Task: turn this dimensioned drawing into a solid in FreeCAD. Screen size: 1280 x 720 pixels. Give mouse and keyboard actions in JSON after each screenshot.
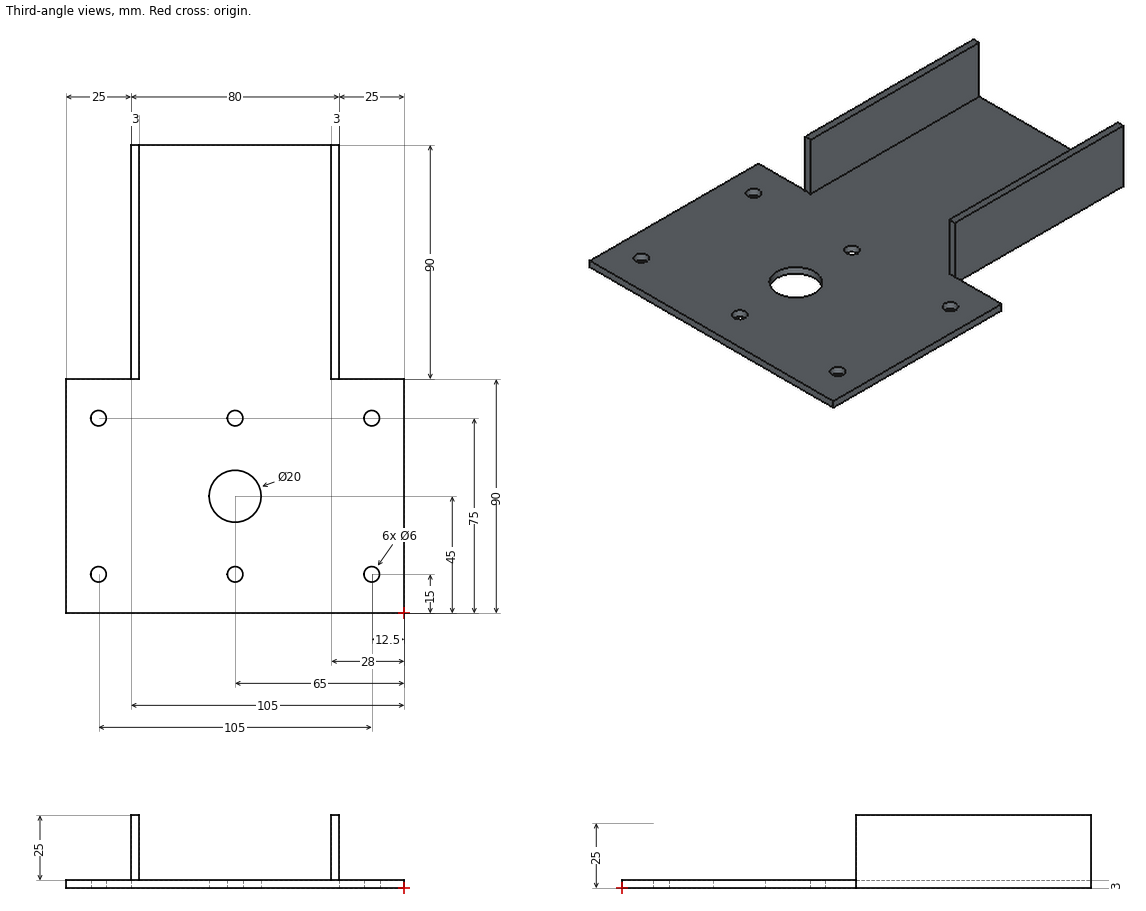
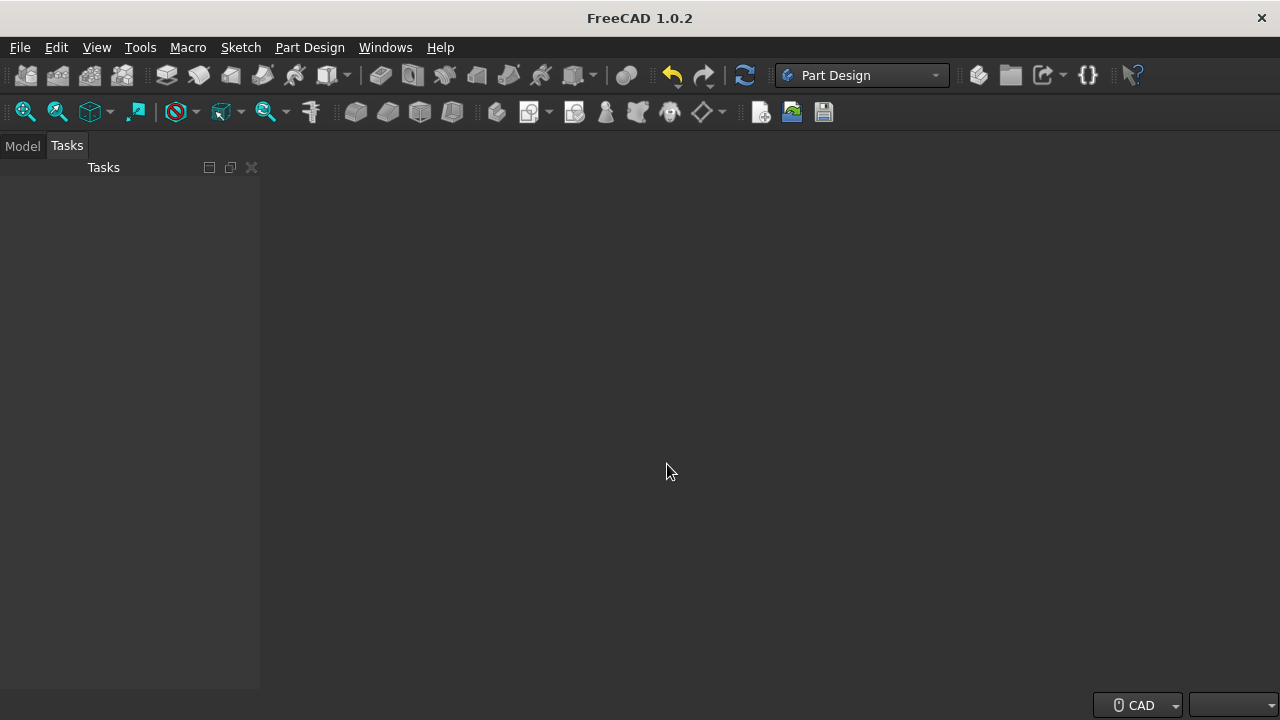
{"action": "left_click", "coordinate": [760, 112]}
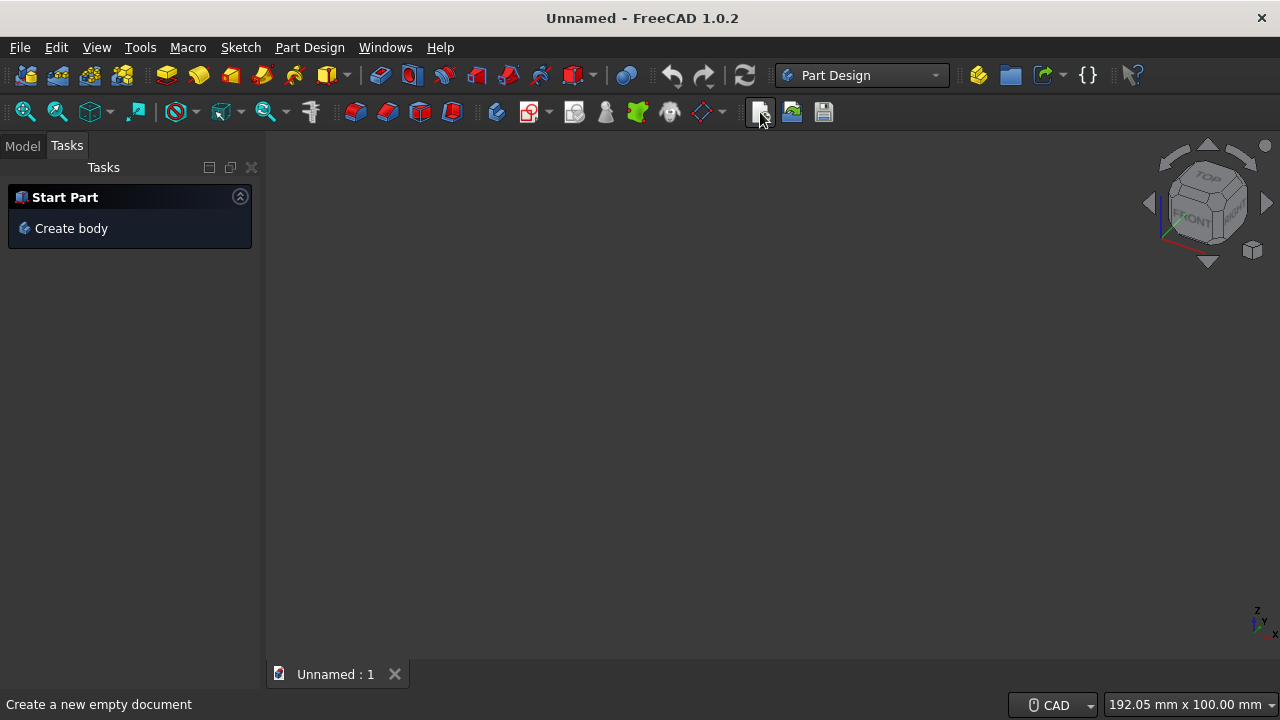
{"action": "left_click", "coordinate": [530, 112]}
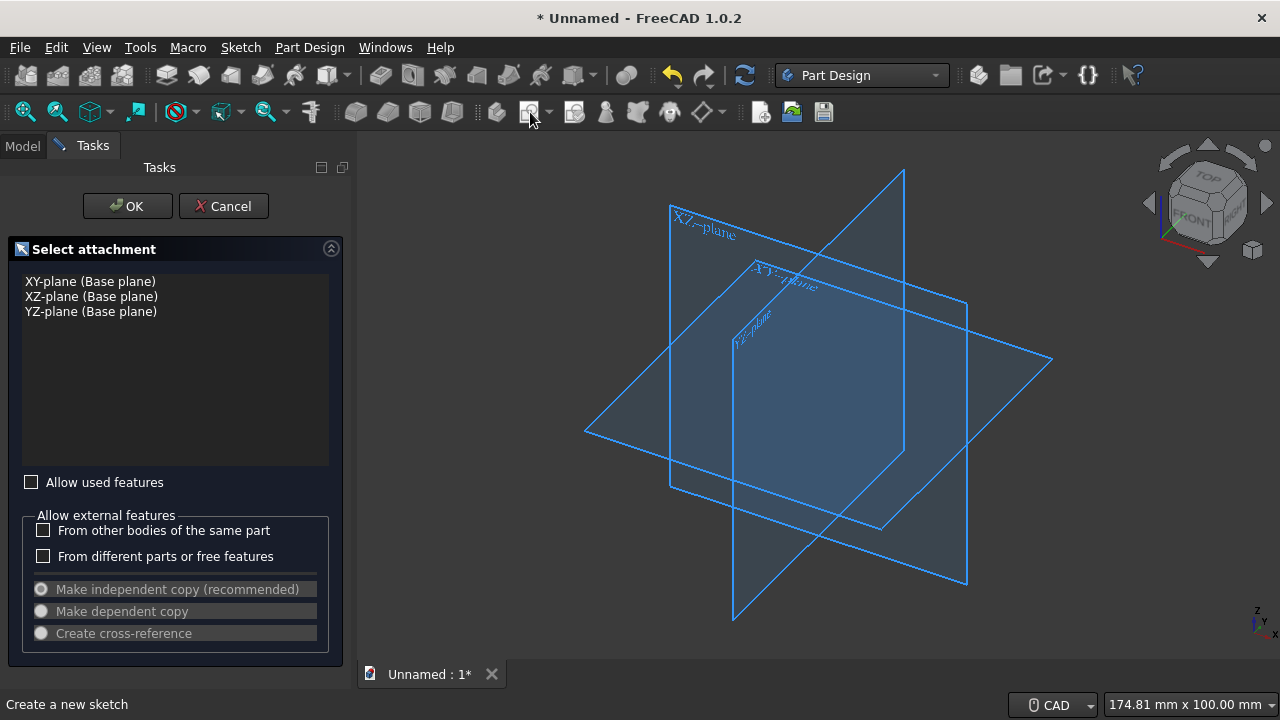
{"action": "left_click", "coordinate": [82, 282]}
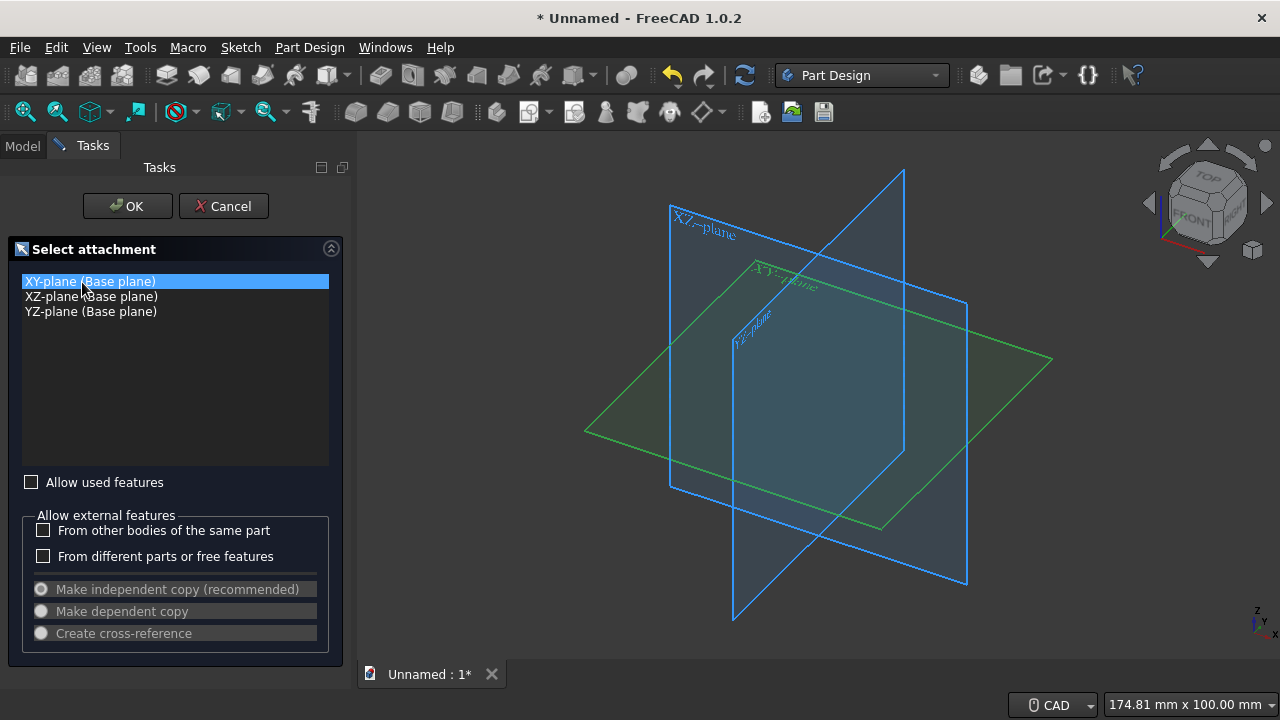
{"action": "left_click", "coordinate": [128, 206]}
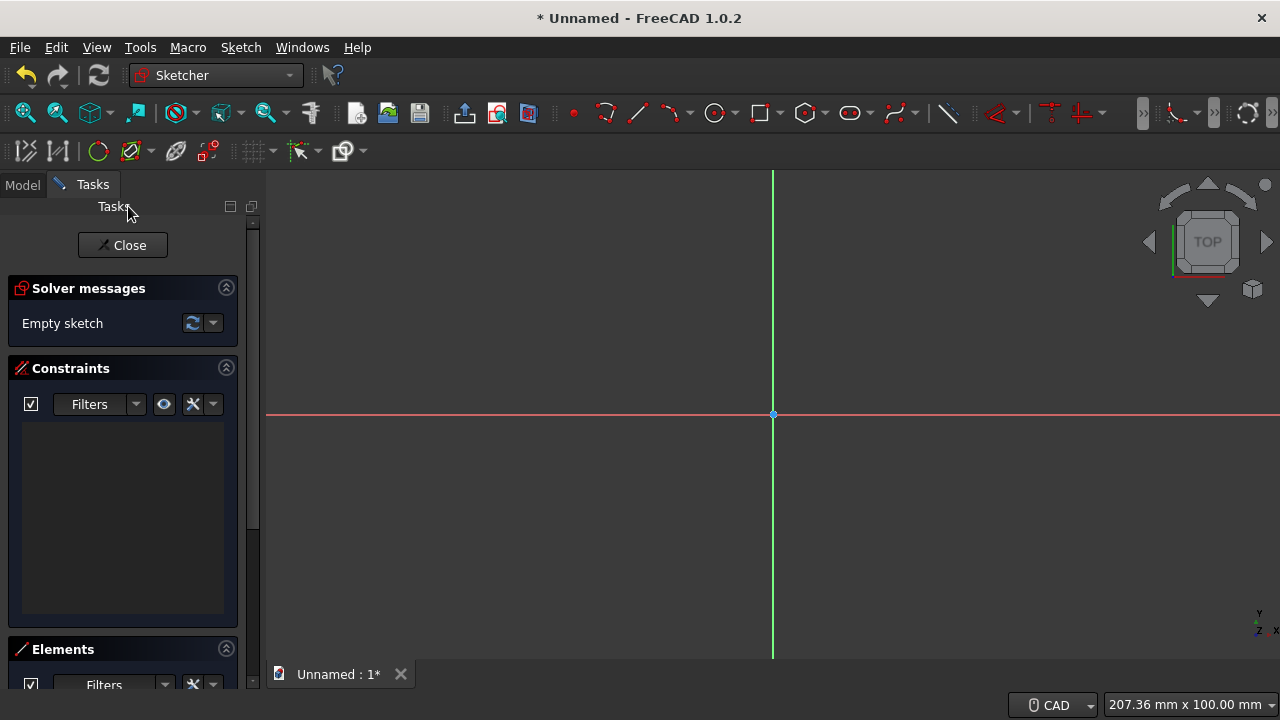
{"action": "scroll", "coordinate": [850, 631], "scroll_direction": "down", "scroll_amount": 5}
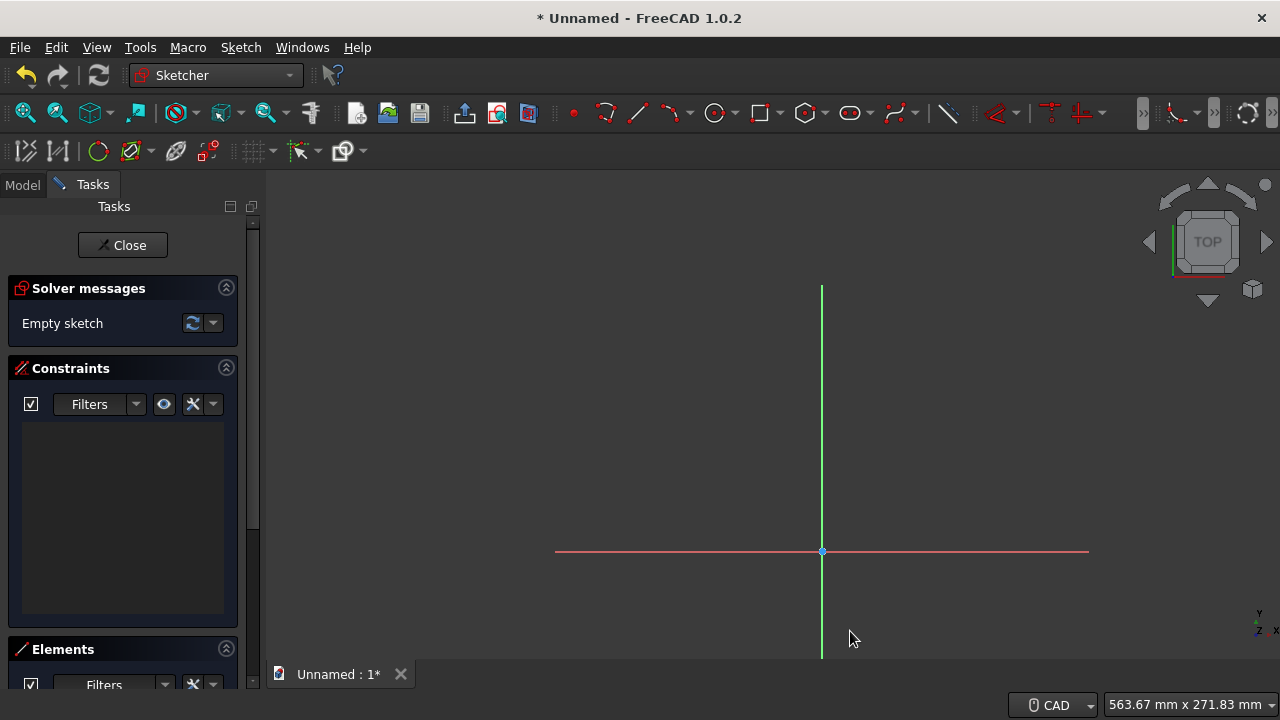
{"action": "left_click", "coordinate": [606, 114]}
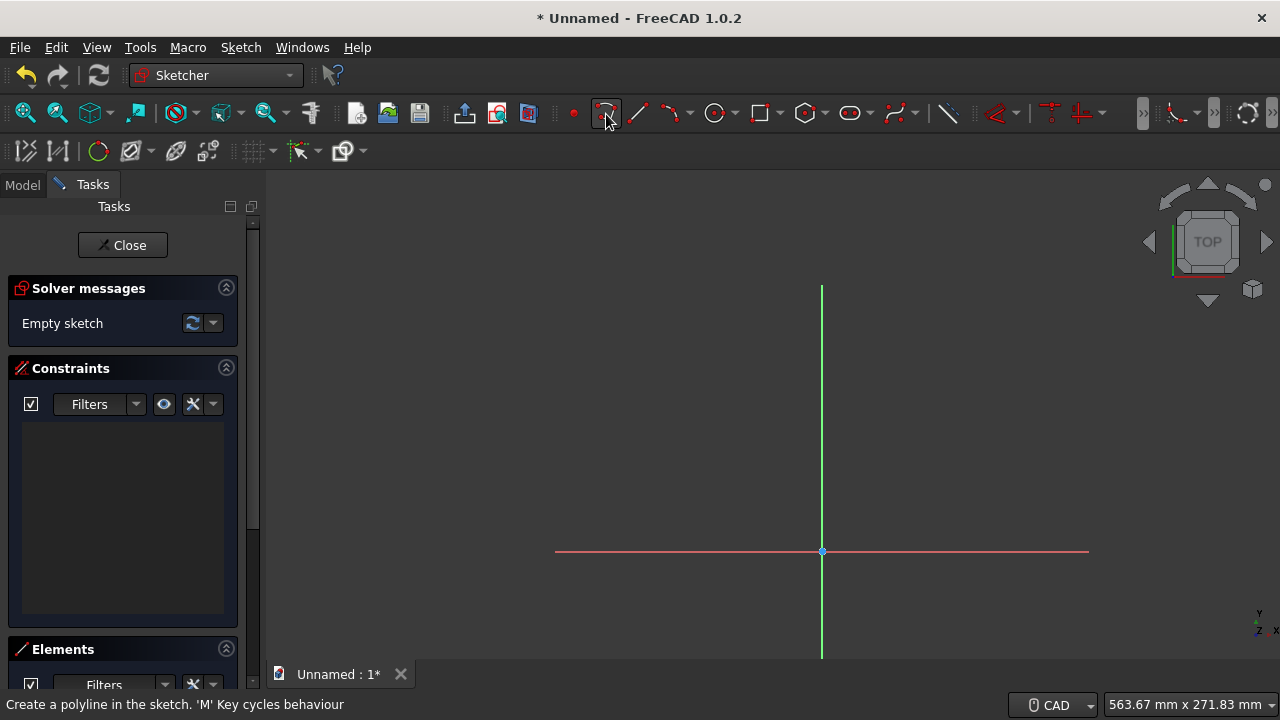
{"action": "left_click", "coordinate": [822, 552]}
{"action": "left_click", "coordinate": [813, 390]}
{"action": "left_click", "coordinate": [777, 390]}
{"action": "left_click", "coordinate": [777, 228]}
{"action": "left_click", "coordinate": [633, 228]}
{"action": "left_click", "coordinate": [633, 390]}
{"action": "left_click", "coordinate": [588, 390]}
{"action": "left_click", "coordinate": [588, 543]}
{"action": "left_click", "coordinate": [822, 552]}
{"action": "key", "text": "Escape"}
{"action": "key", "text": "Escape"}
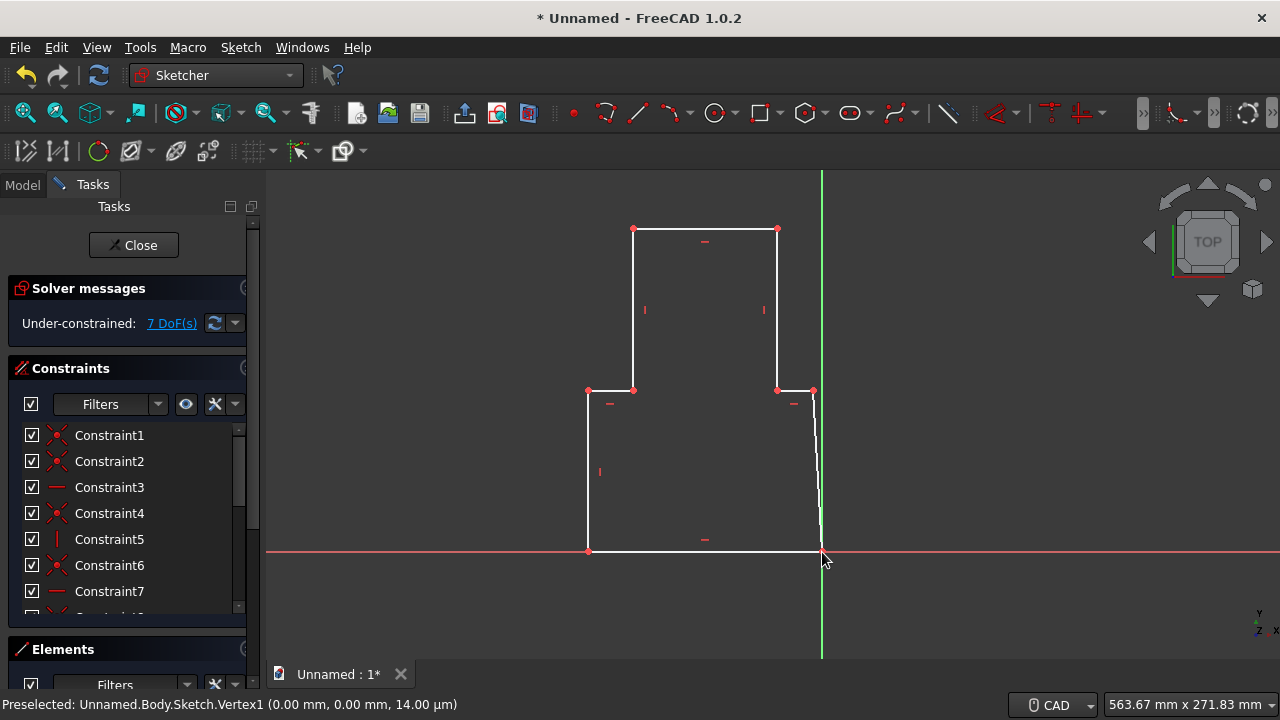
{"action": "left_click", "coordinate": [819, 504]}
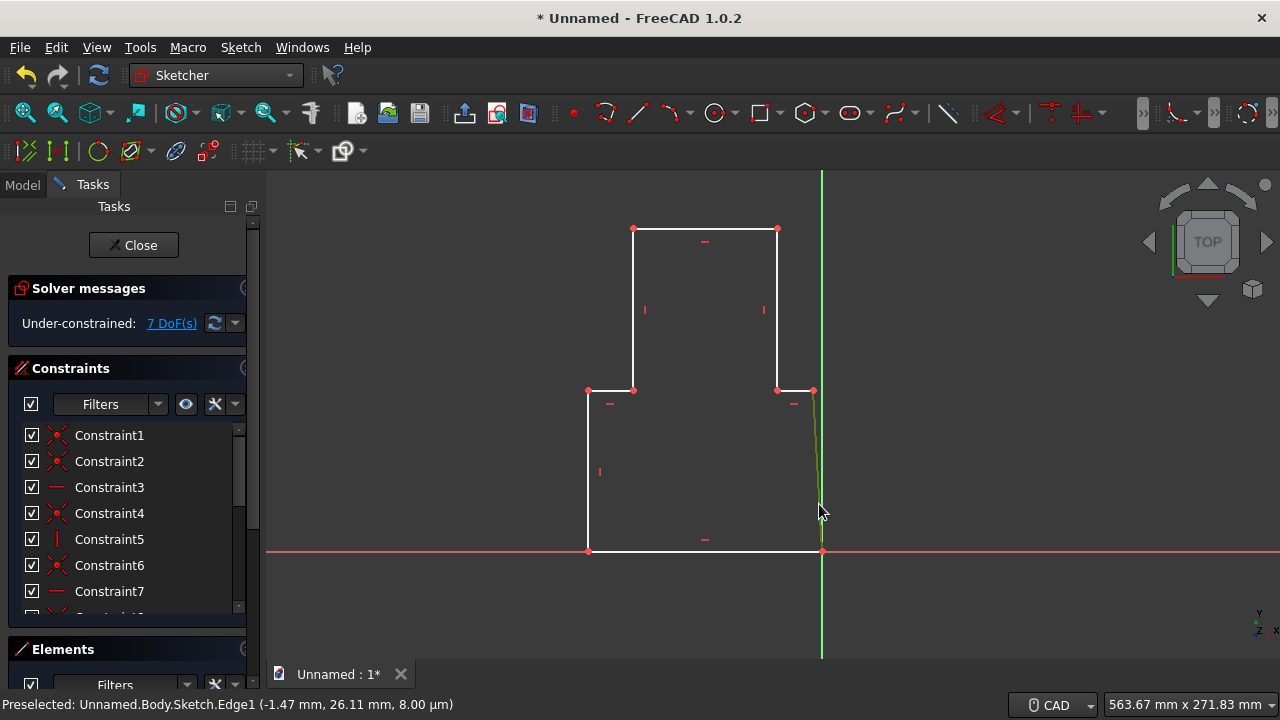
{"action": "key", "text": "v"}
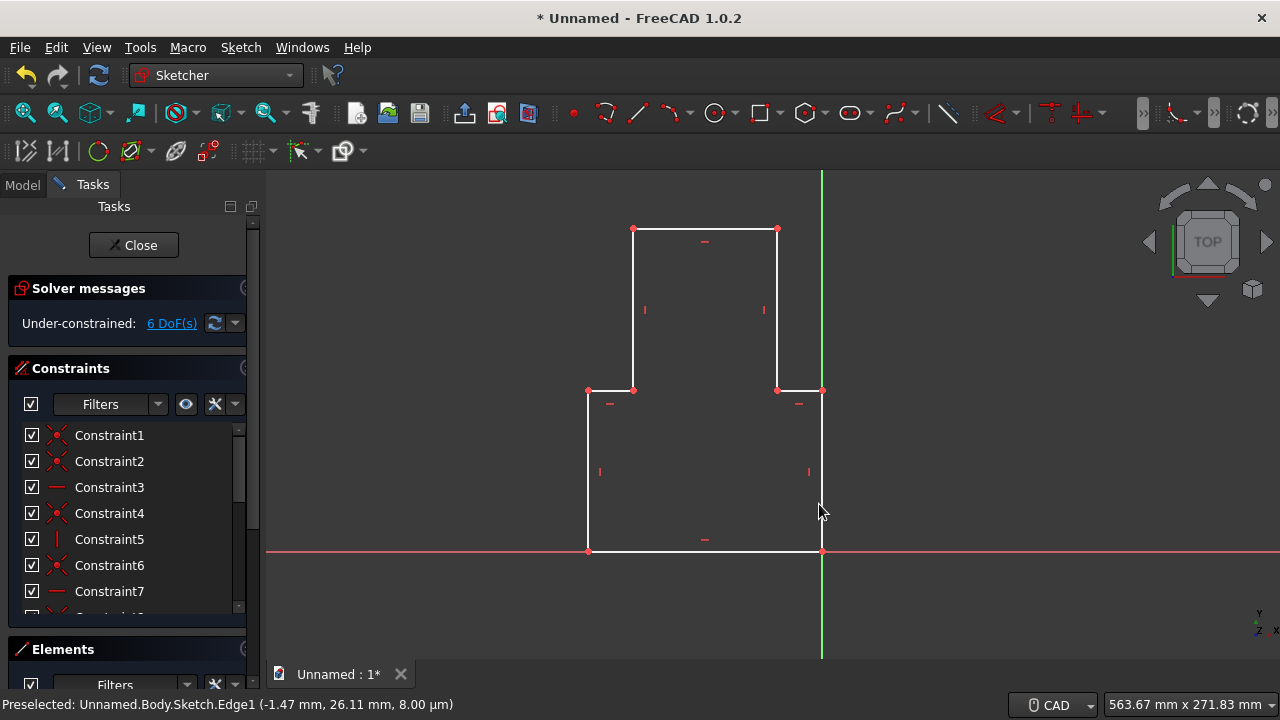
{"action": "key", "text": "d"}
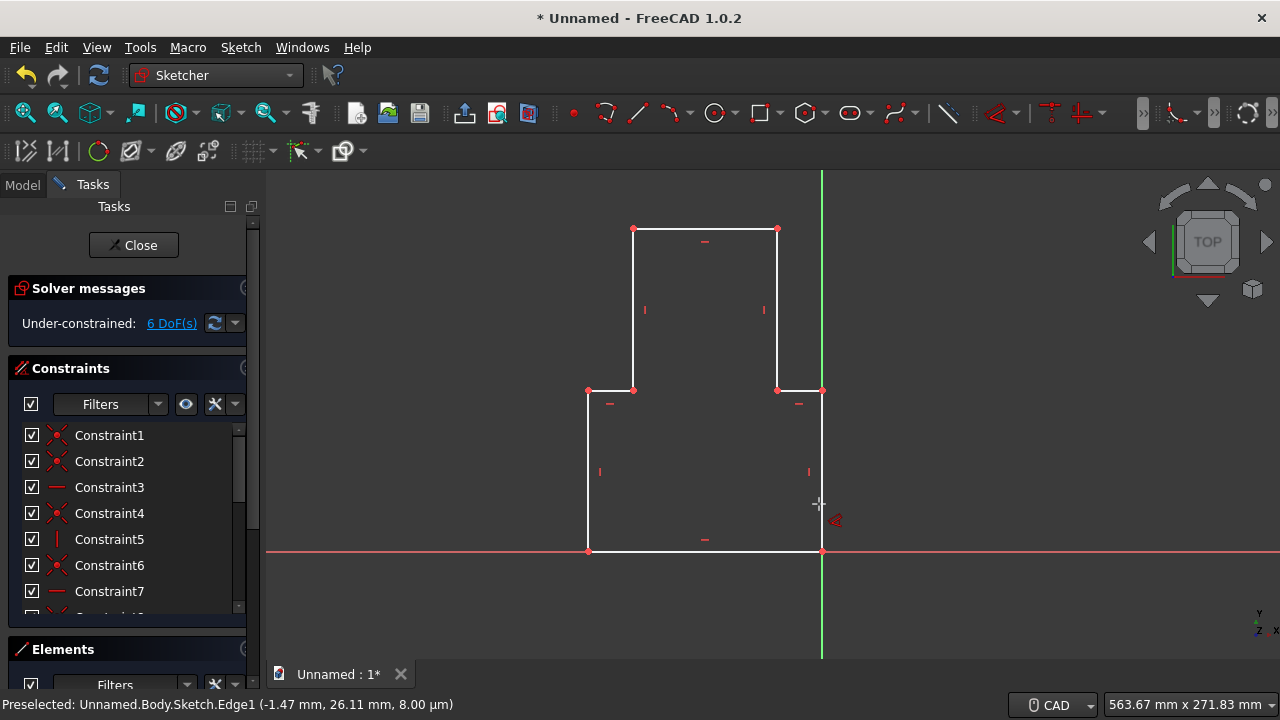
{"action": "left_click", "coordinate": [822, 504]}
{"action": "left_click", "coordinate": [856, 471]}